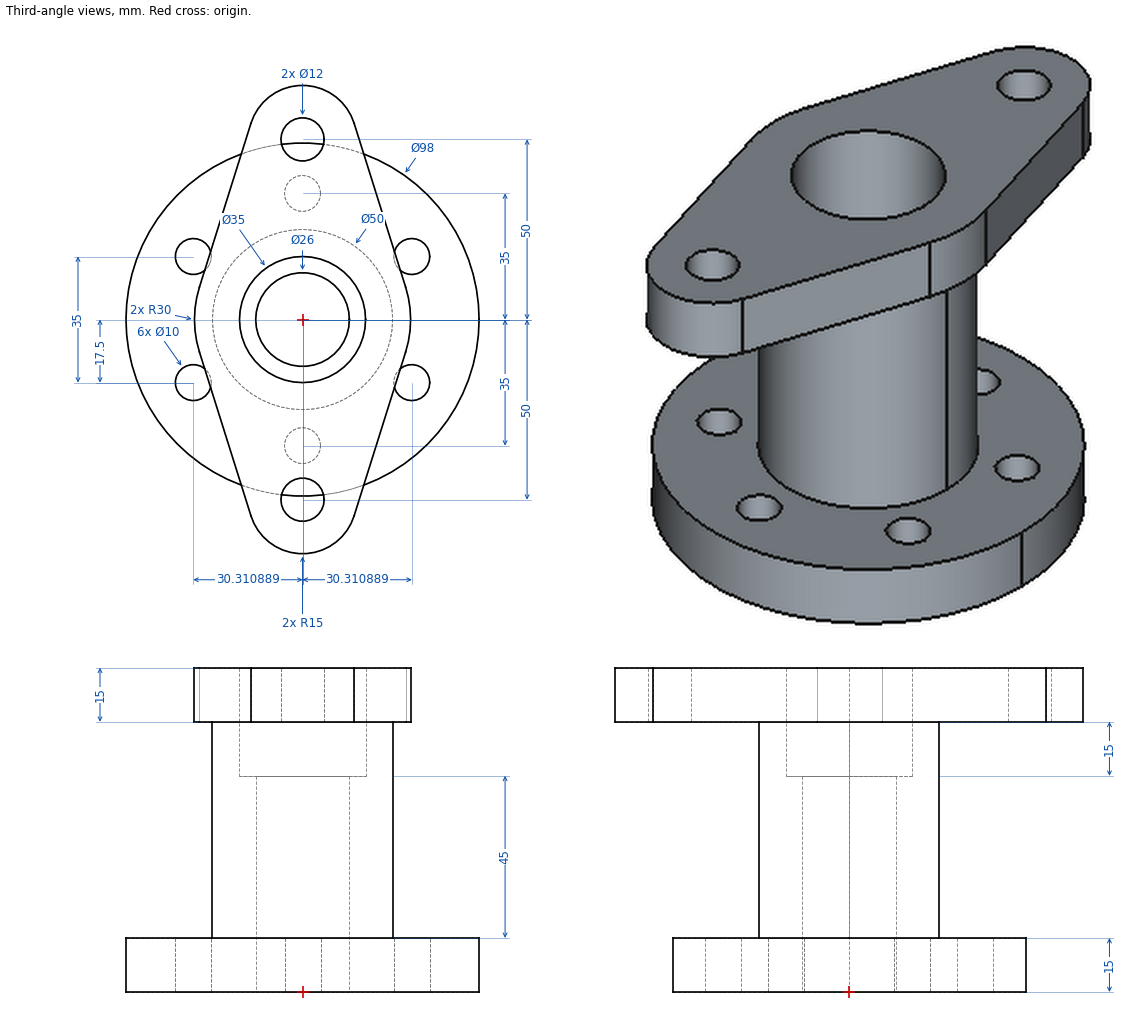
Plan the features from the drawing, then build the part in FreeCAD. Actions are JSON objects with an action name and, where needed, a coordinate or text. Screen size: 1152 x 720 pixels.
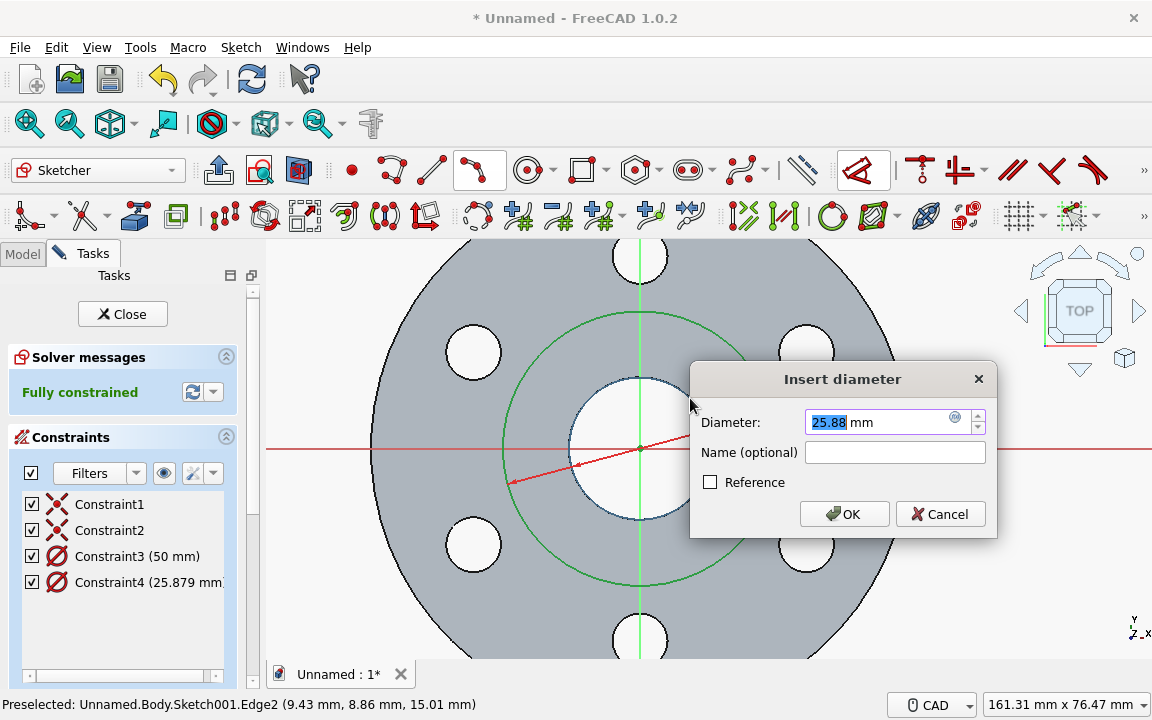
{"action": "type", "text": "26"}
{"action": "key", "text": "Return"}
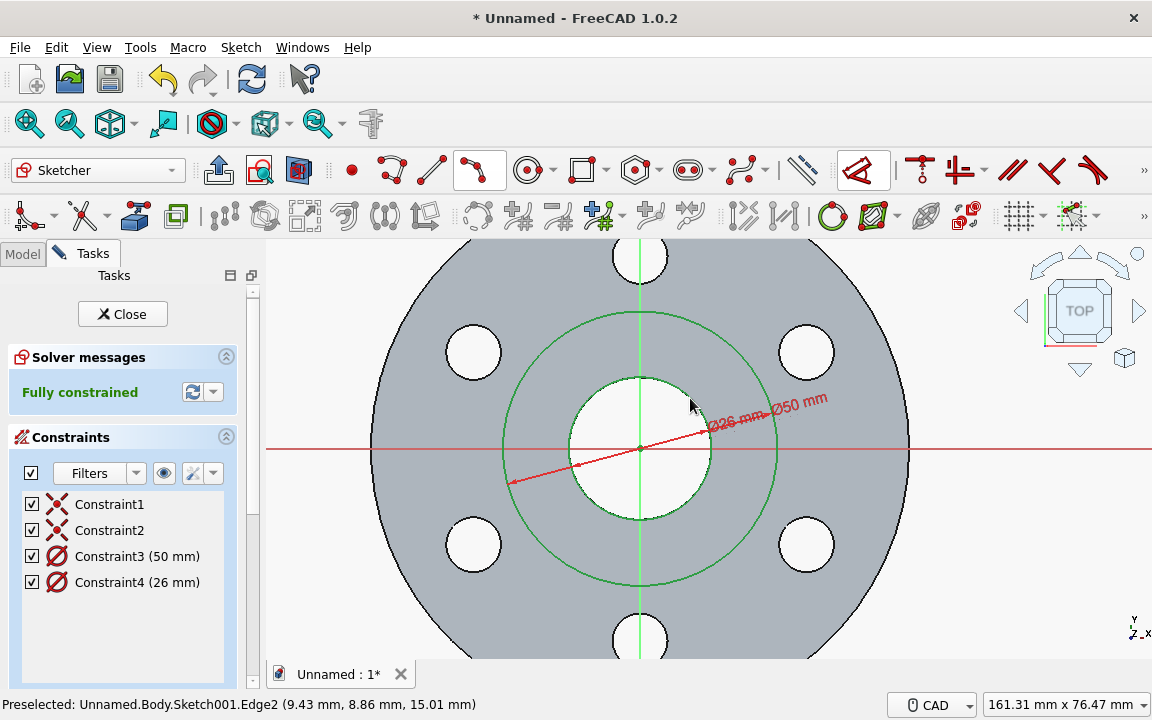
{"action": "left_click", "coordinate": [123, 314]}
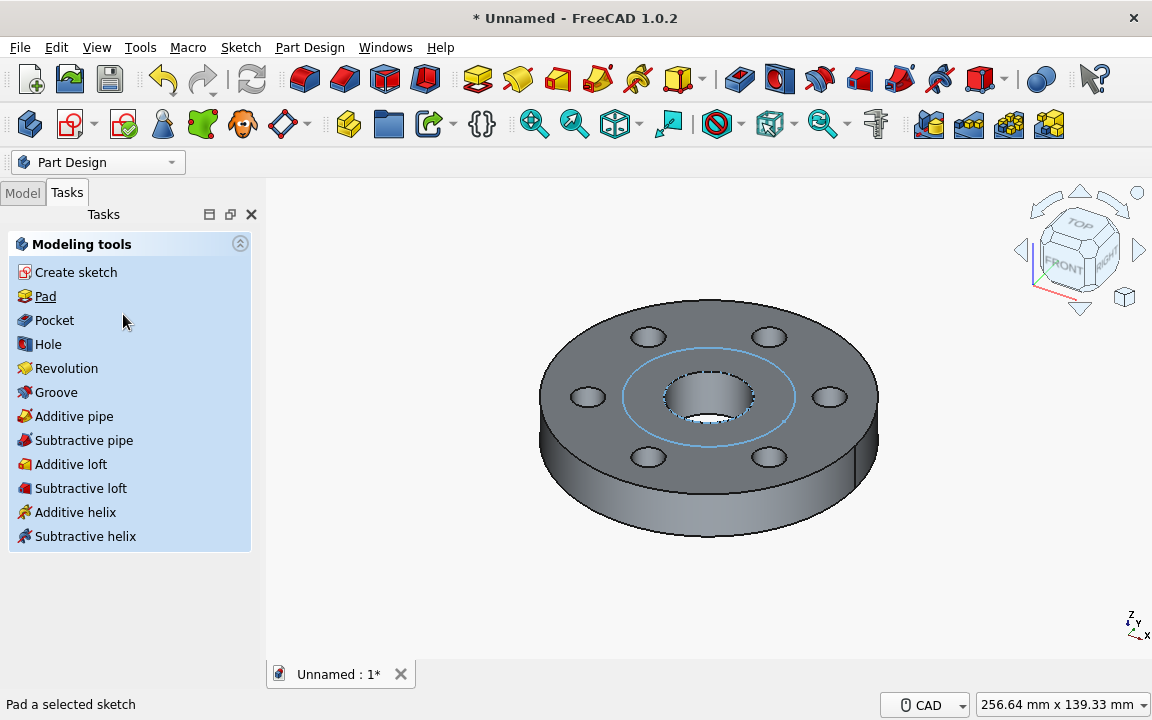
{"action": "left_click", "coordinate": [478, 80]}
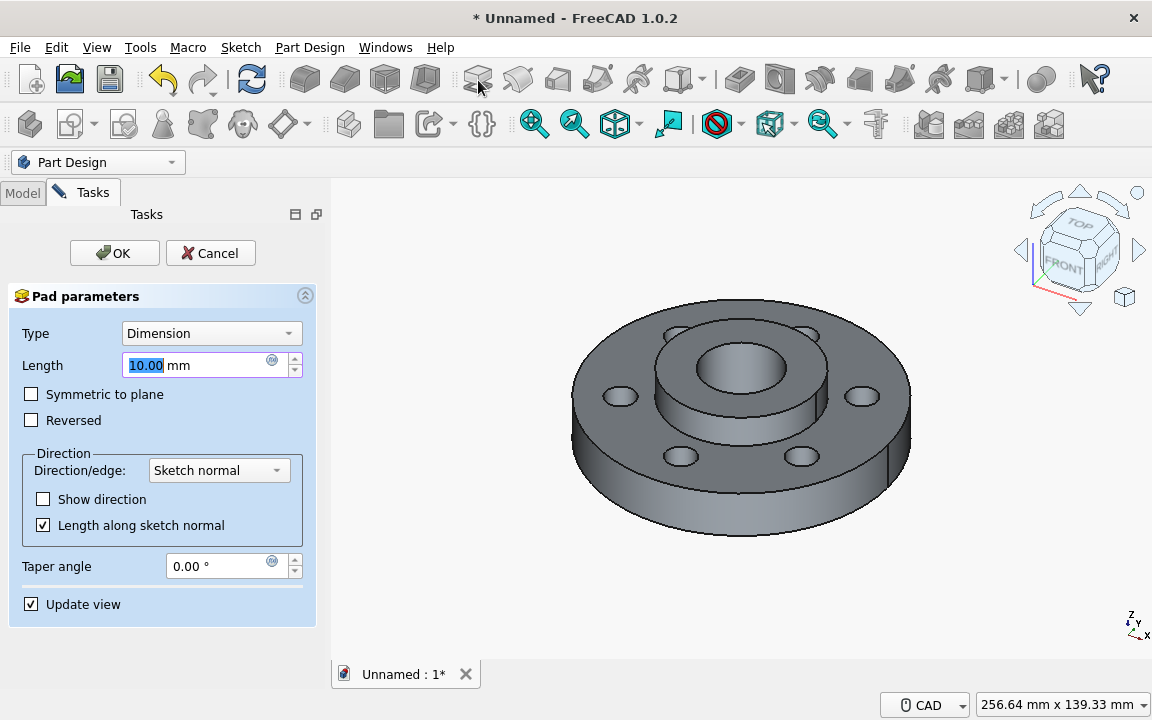
{"action": "type", "text": "45"}
{"action": "key", "text": "Tab"}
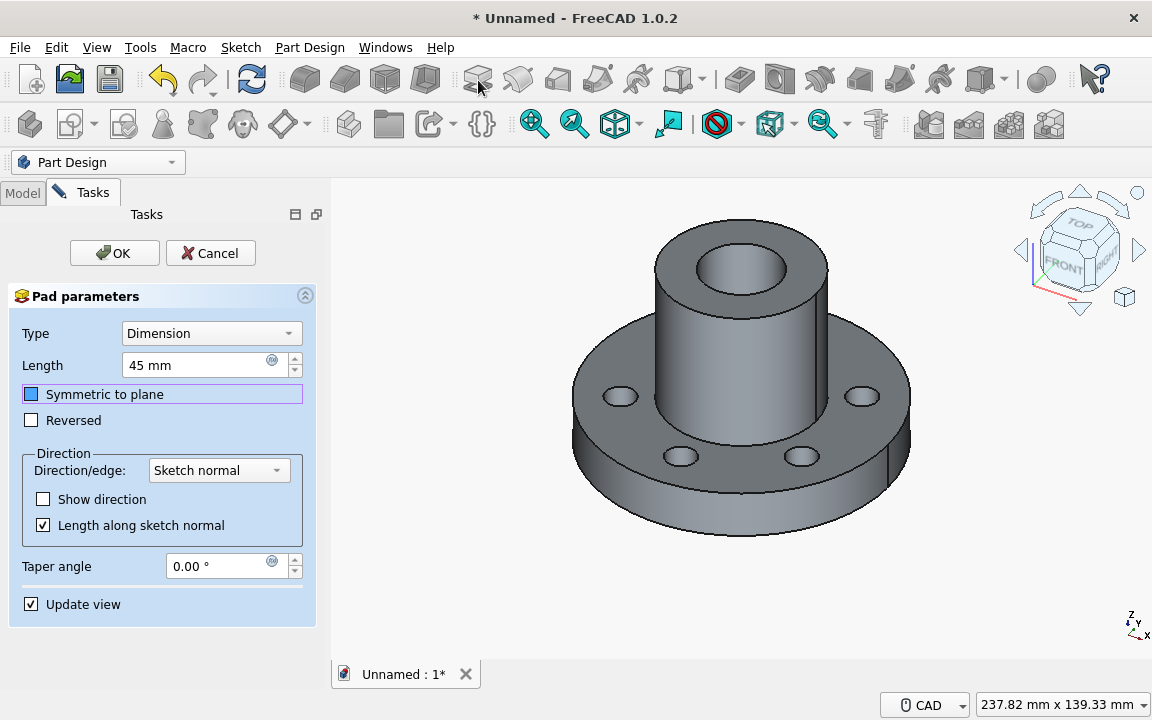
{"action": "left_click", "coordinate": [115, 253]}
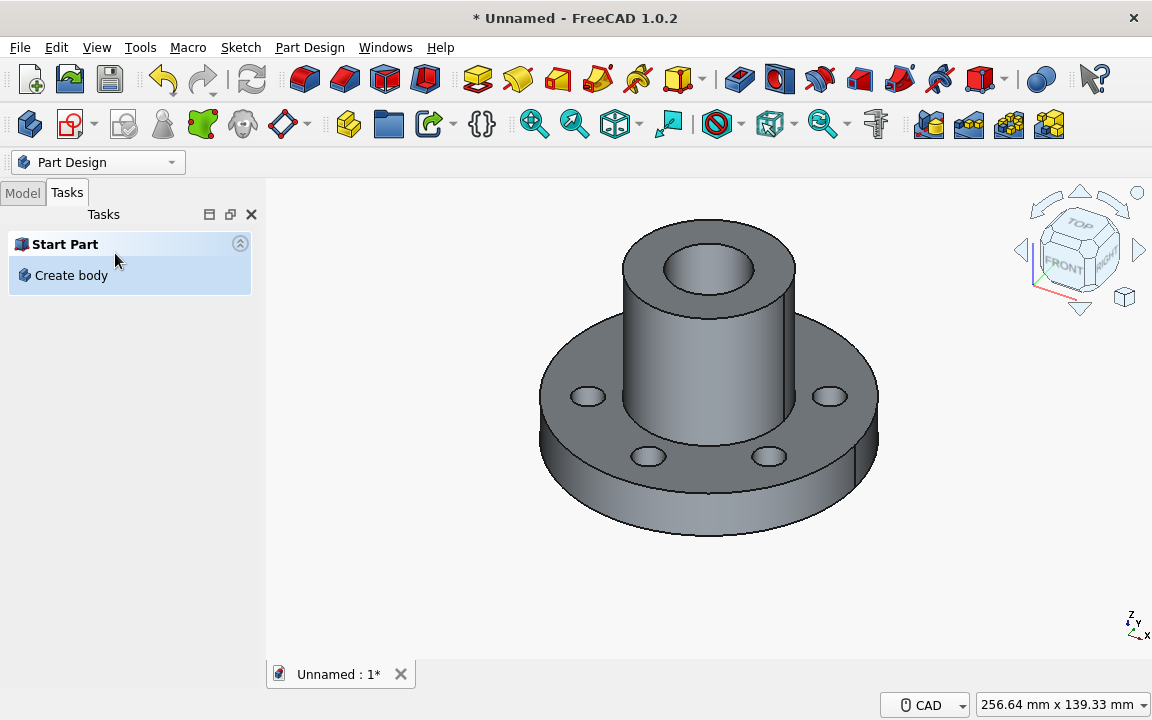
{"action": "left_click", "coordinate": [536, 124]}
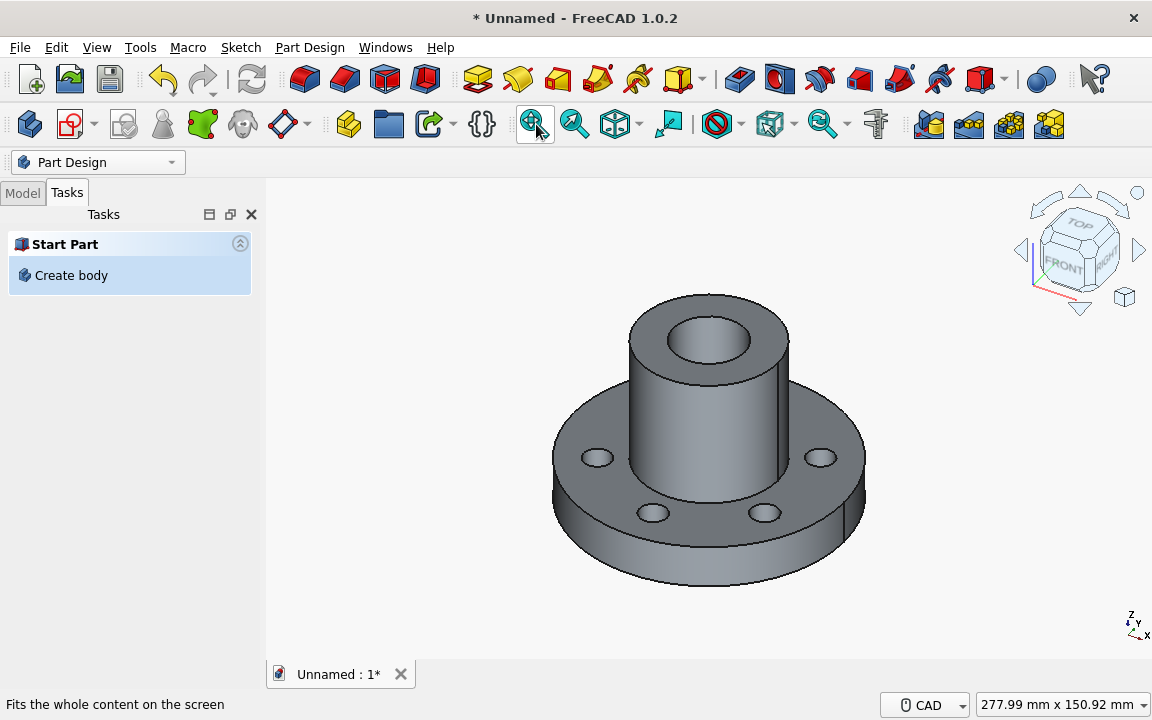
{"action": "left_click", "coordinate": [726, 375]}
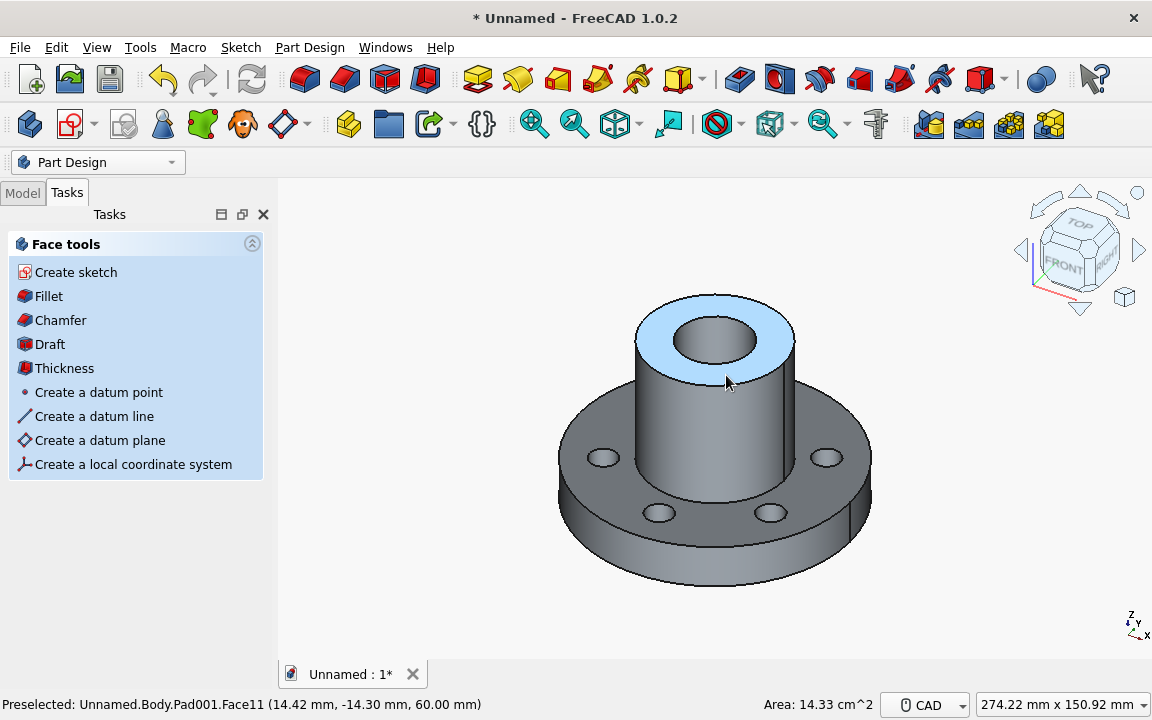
{"action": "left_click", "coordinate": [70, 124]}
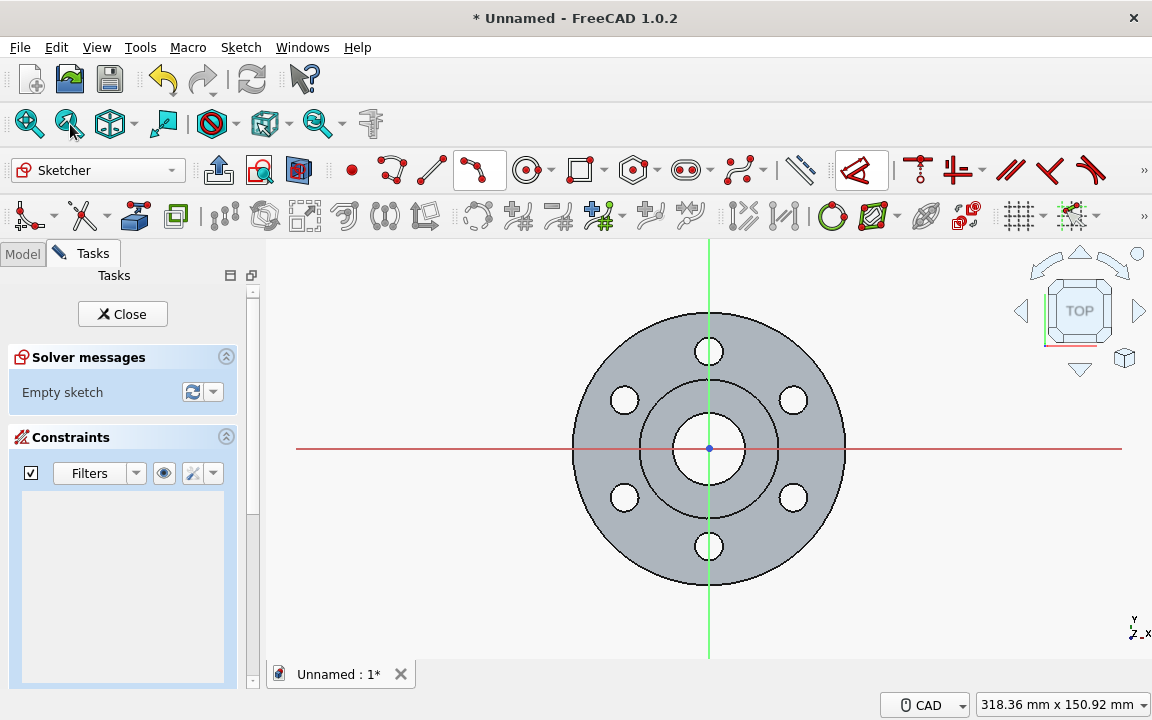
{"action": "scroll", "coordinate": [792, 449], "scroll_direction": "up", "scroll_amount": 3}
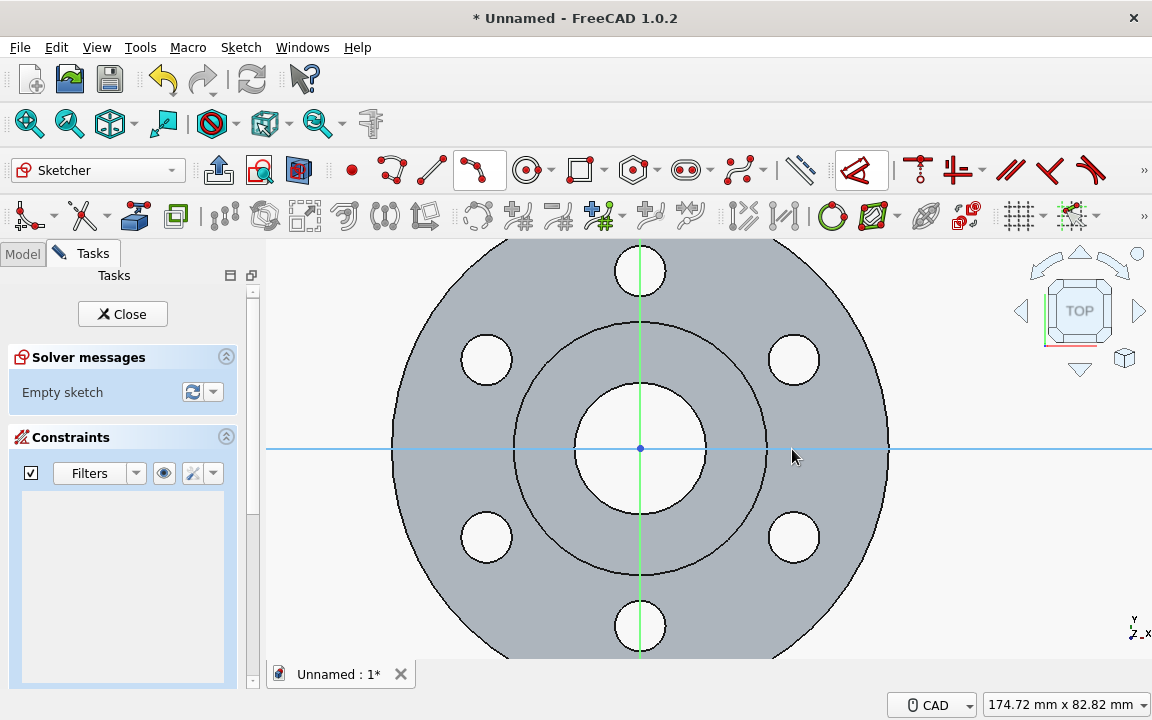
{"action": "key", "text": "g c"}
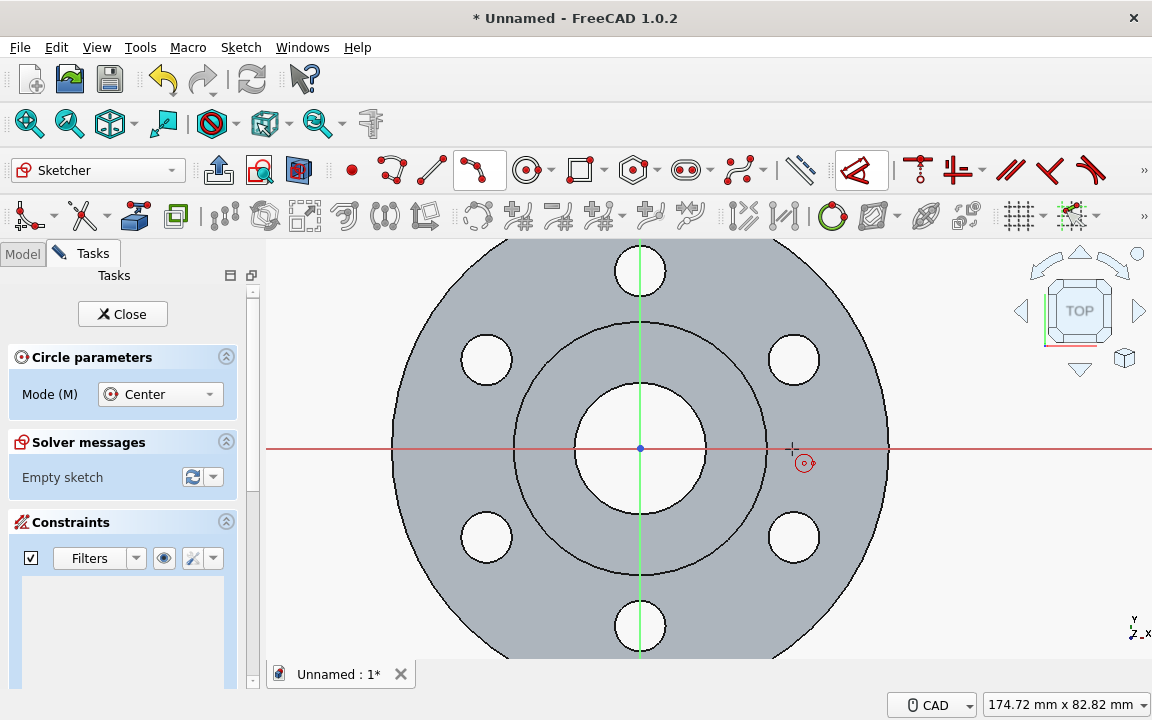
{"action": "left_click", "coordinate": [640, 449]}
{"action": "left_click", "coordinate": [730, 359]}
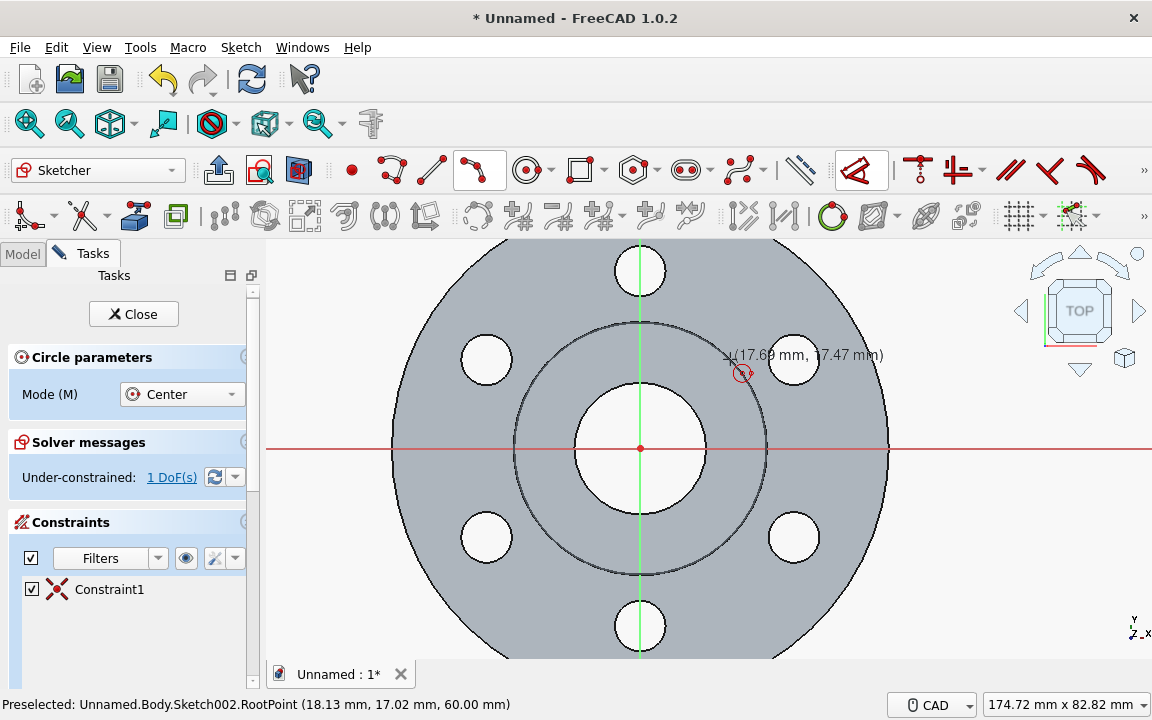
{"action": "left_click", "coordinate": [640, 449]}
{"action": "left_click", "coordinate": [703, 386]}
{"action": "key", "text": "Escape"}